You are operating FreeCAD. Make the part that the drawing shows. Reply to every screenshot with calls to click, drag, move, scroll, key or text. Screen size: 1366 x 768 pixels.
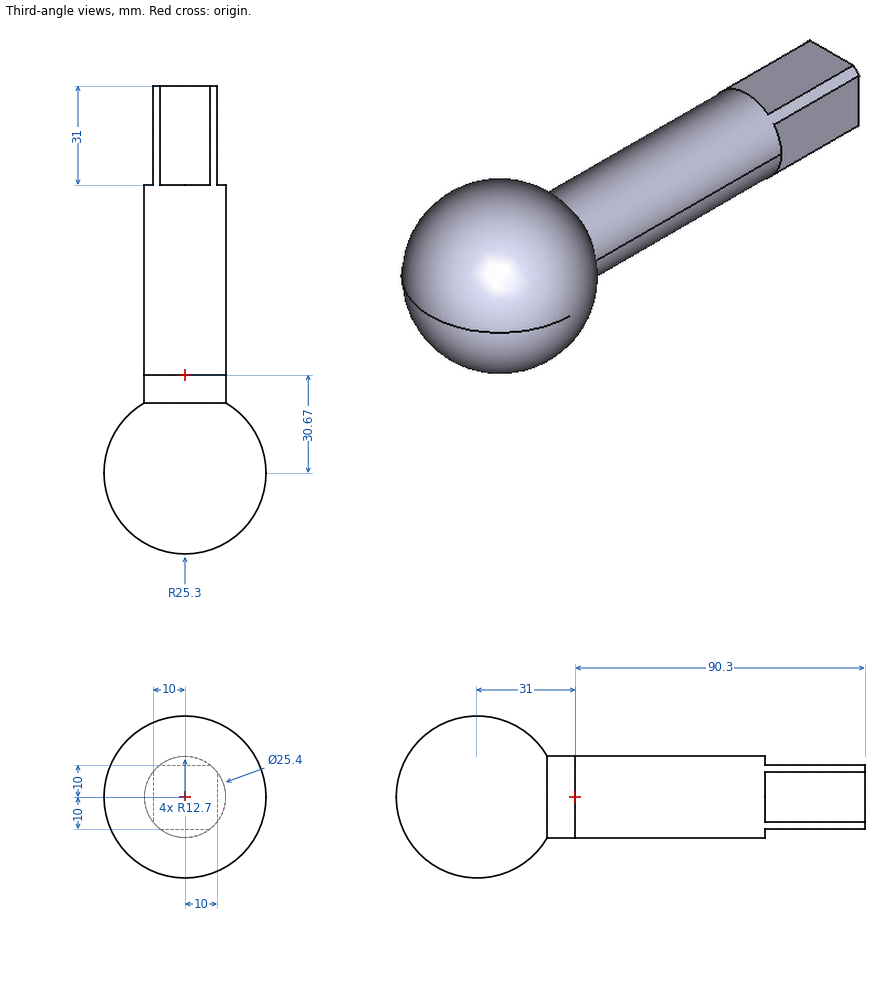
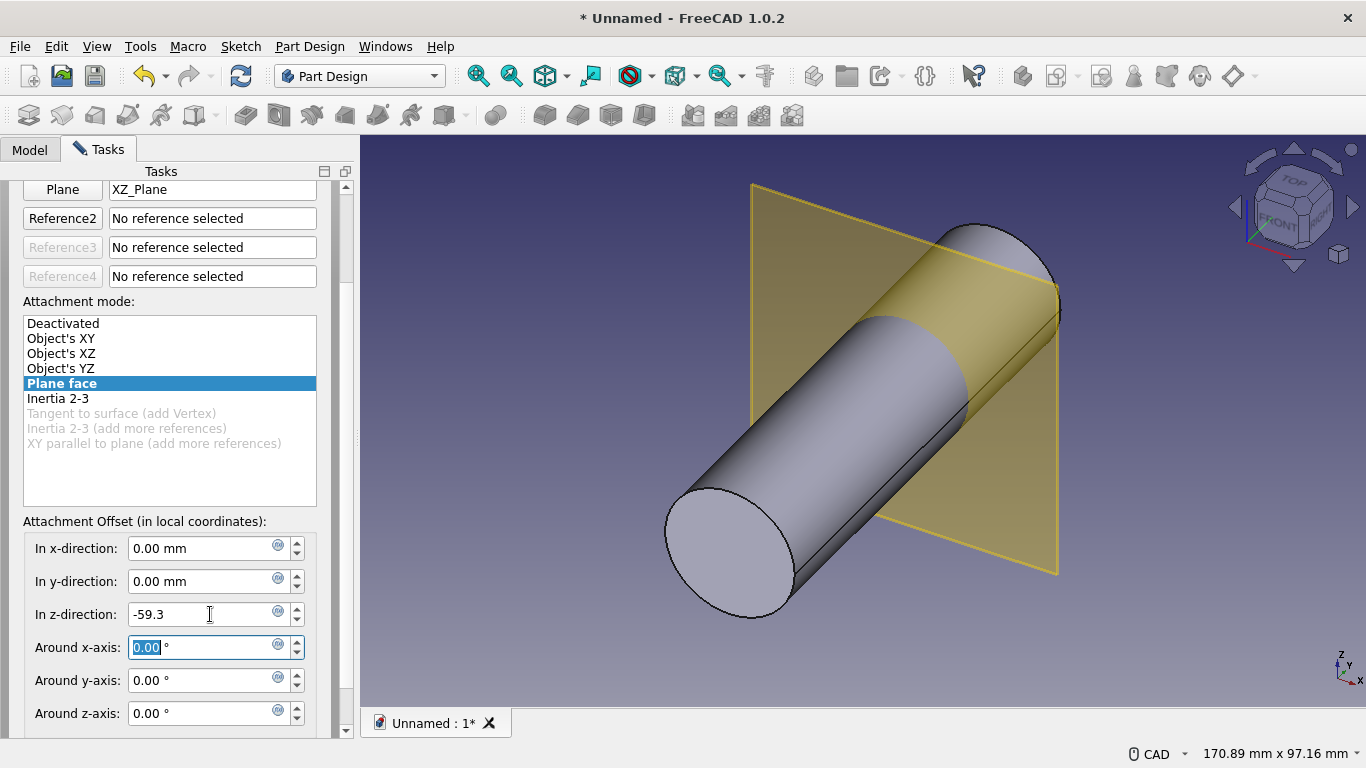
scroll(346, 460, up, 3)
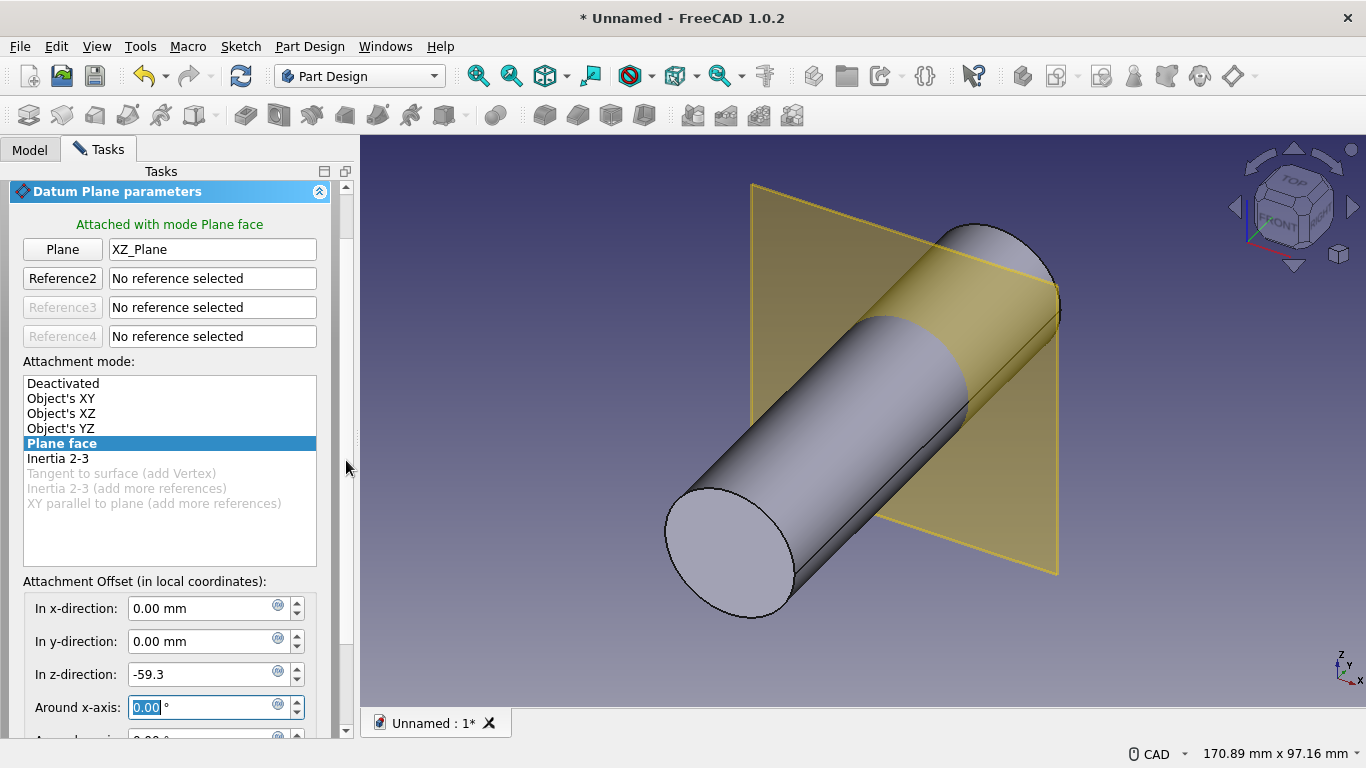
click(127, 210)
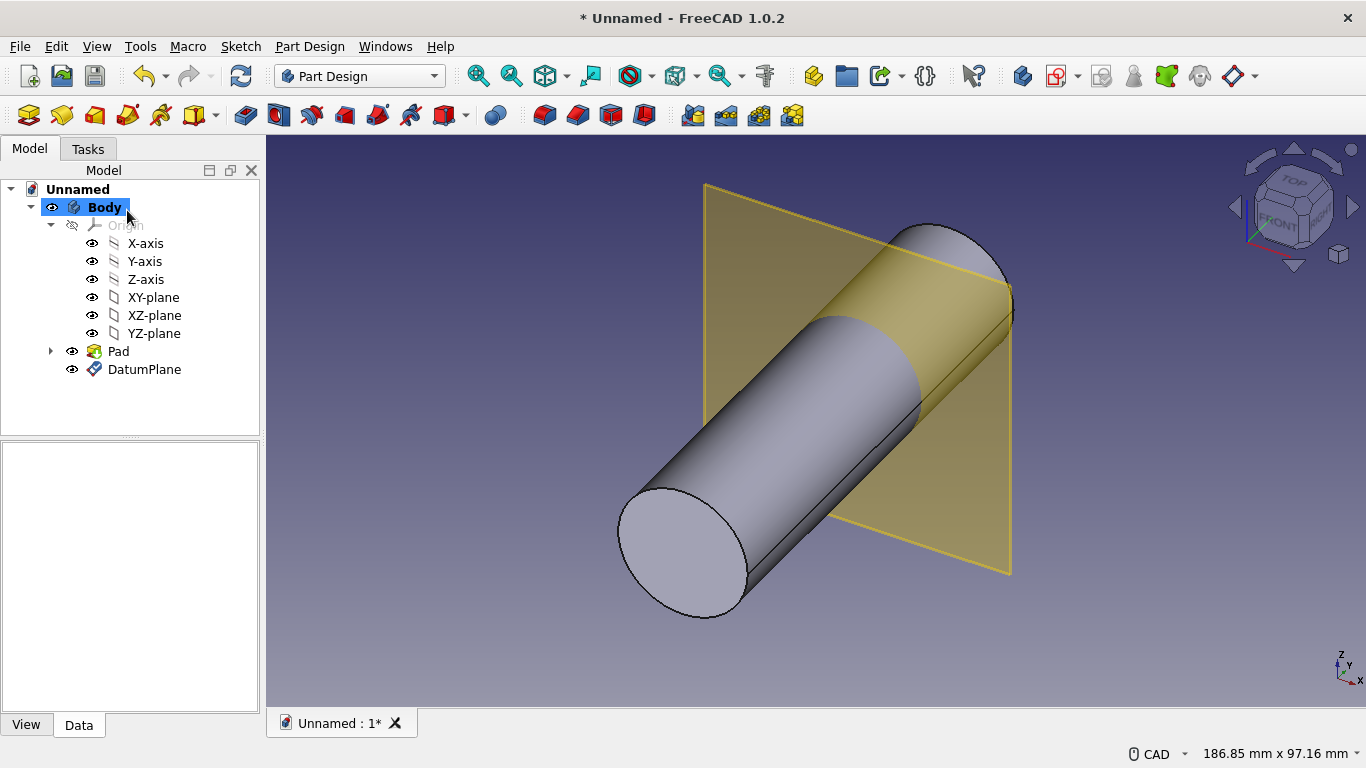
click(117, 369)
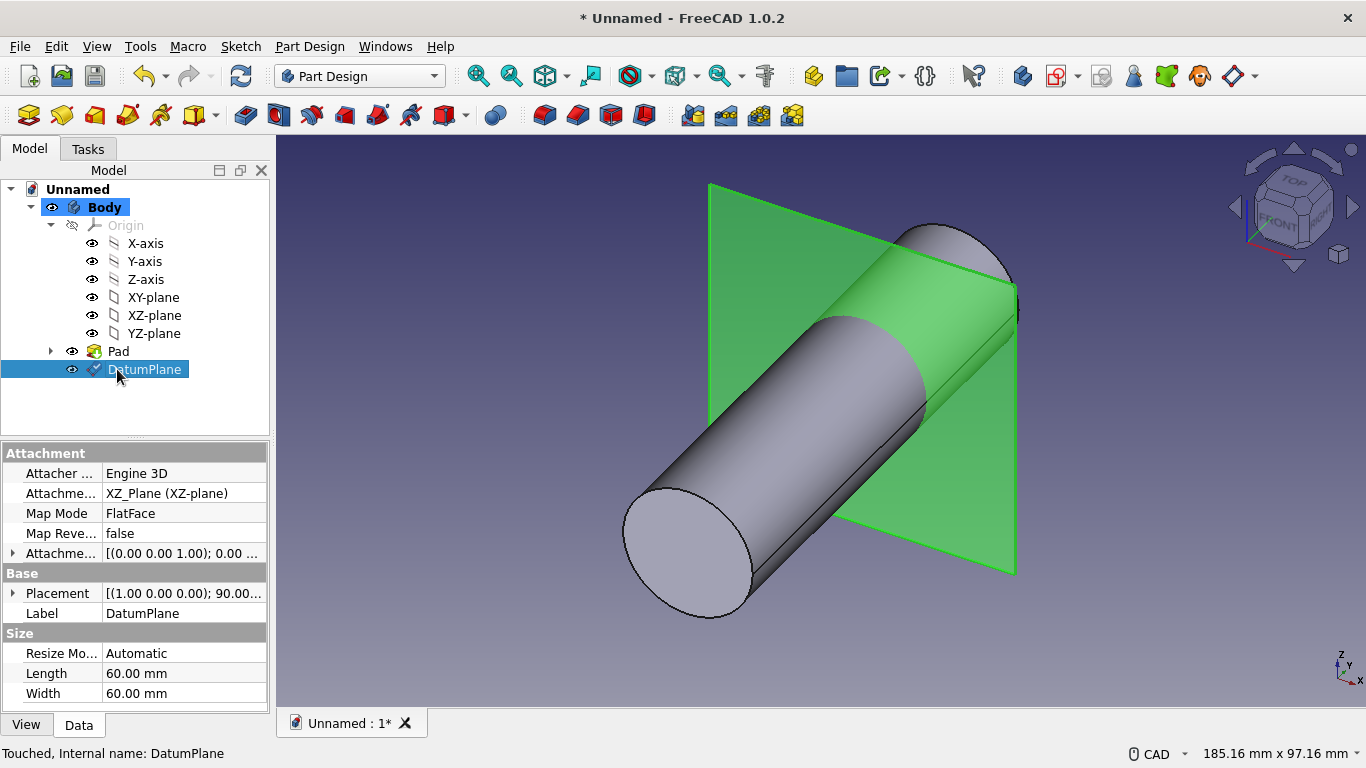
click(1056, 76)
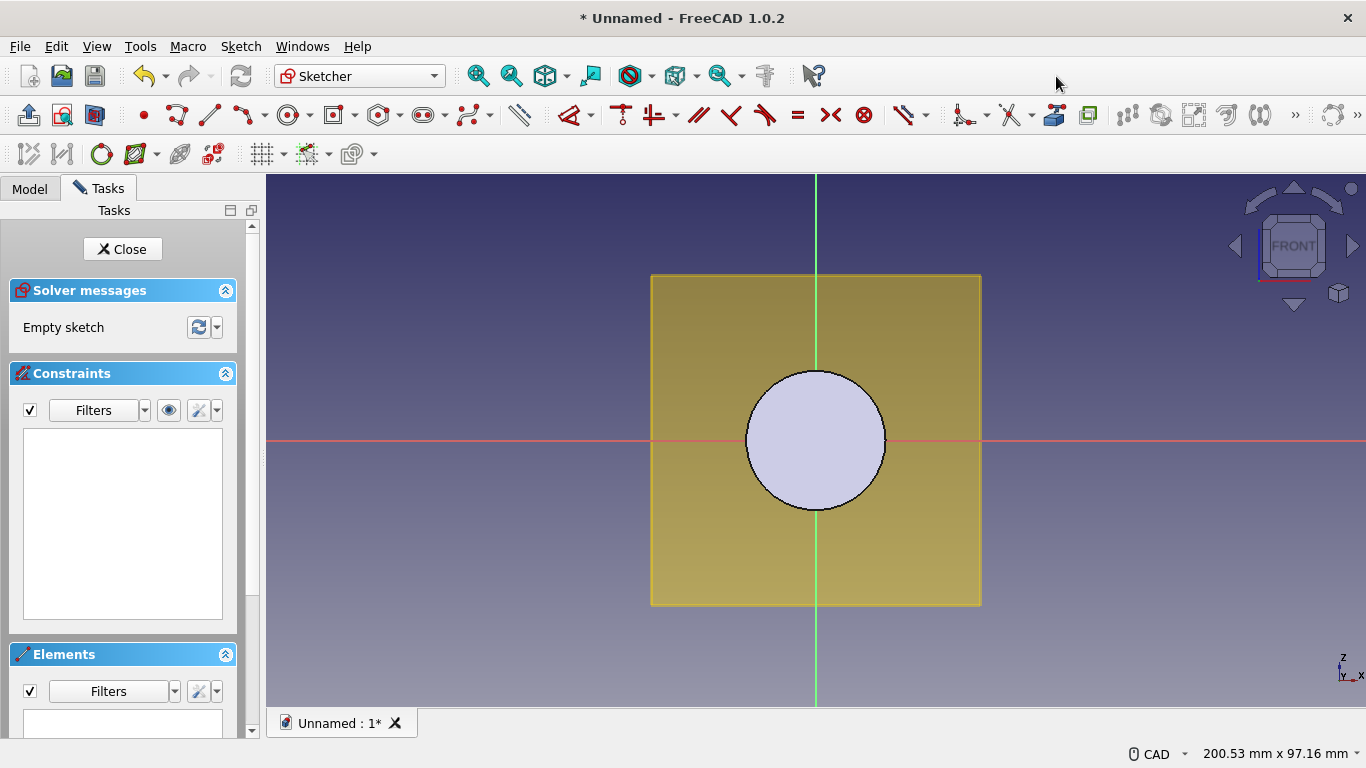
key(q)
key(s)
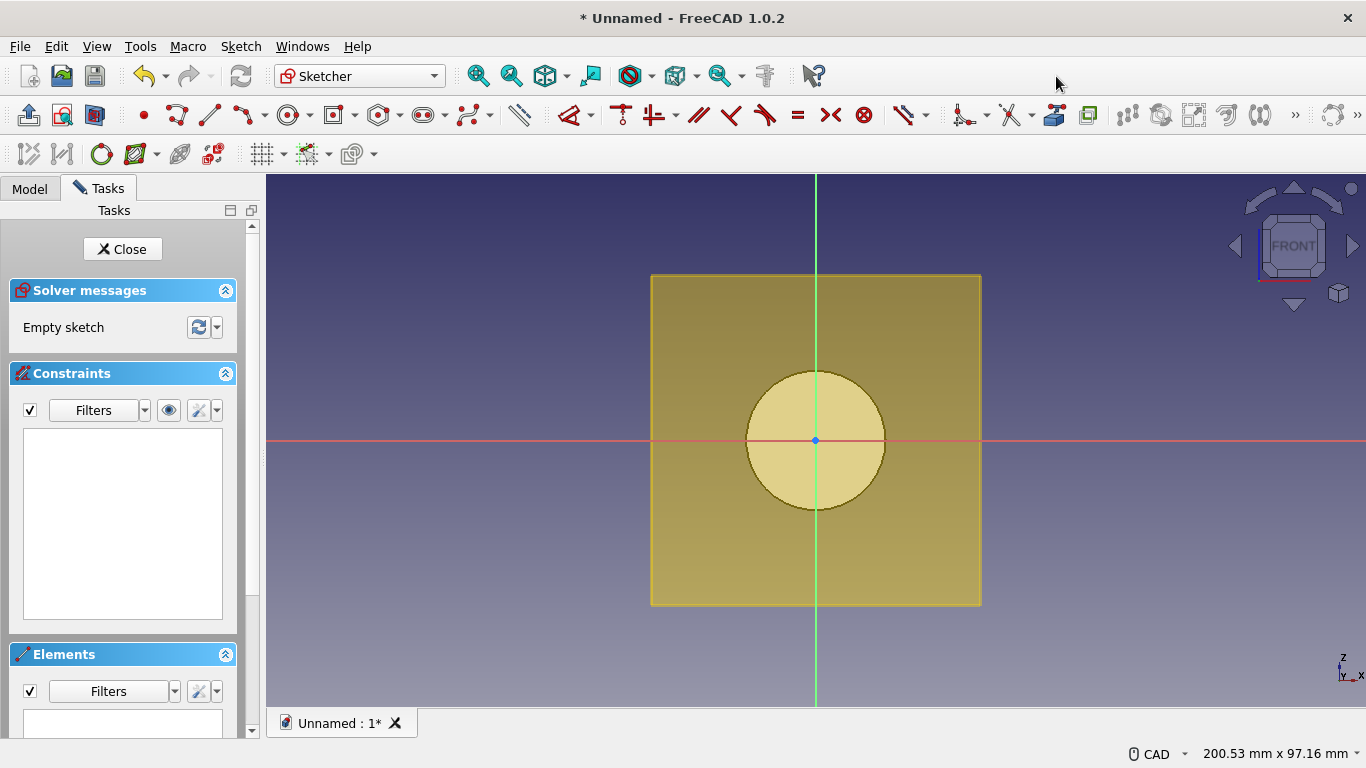
scroll(872, 441, up, 4)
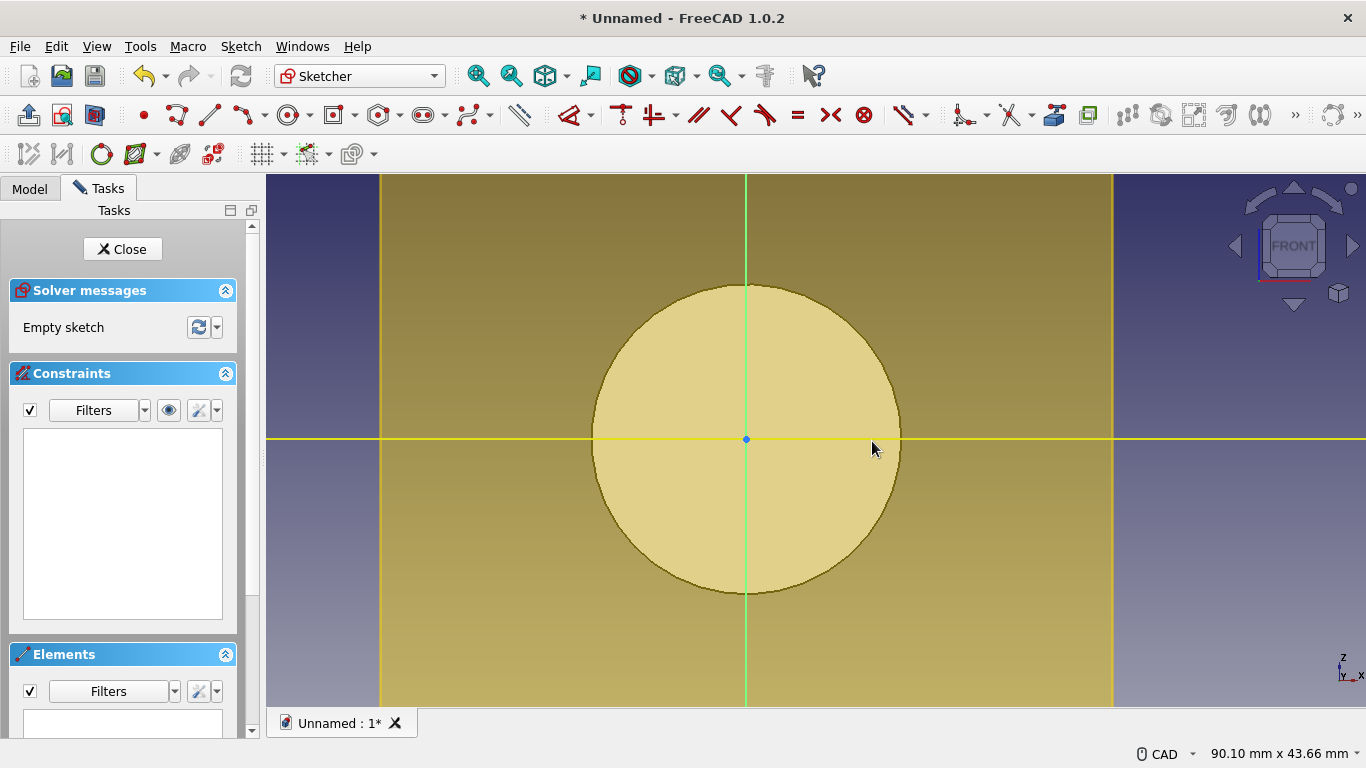
click(210, 116)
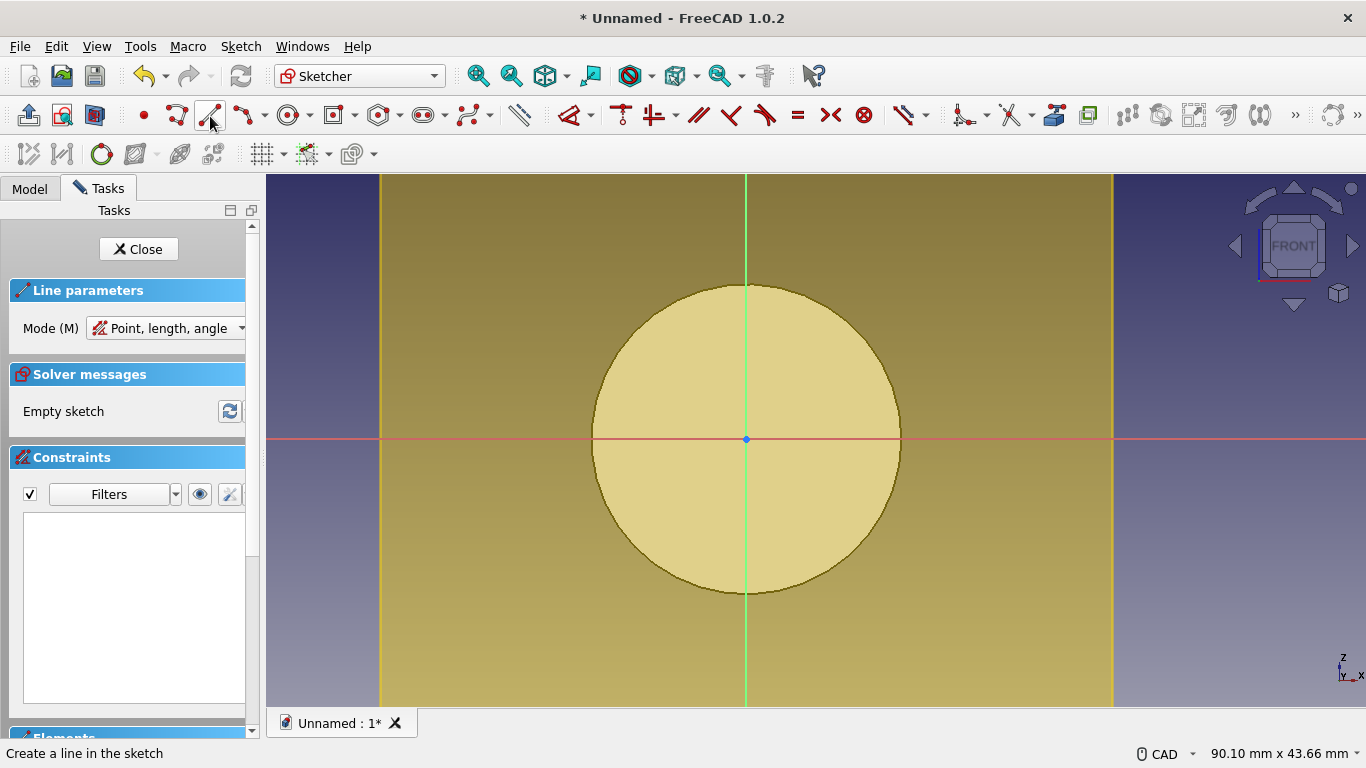
click(651, 317)
click(842, 317)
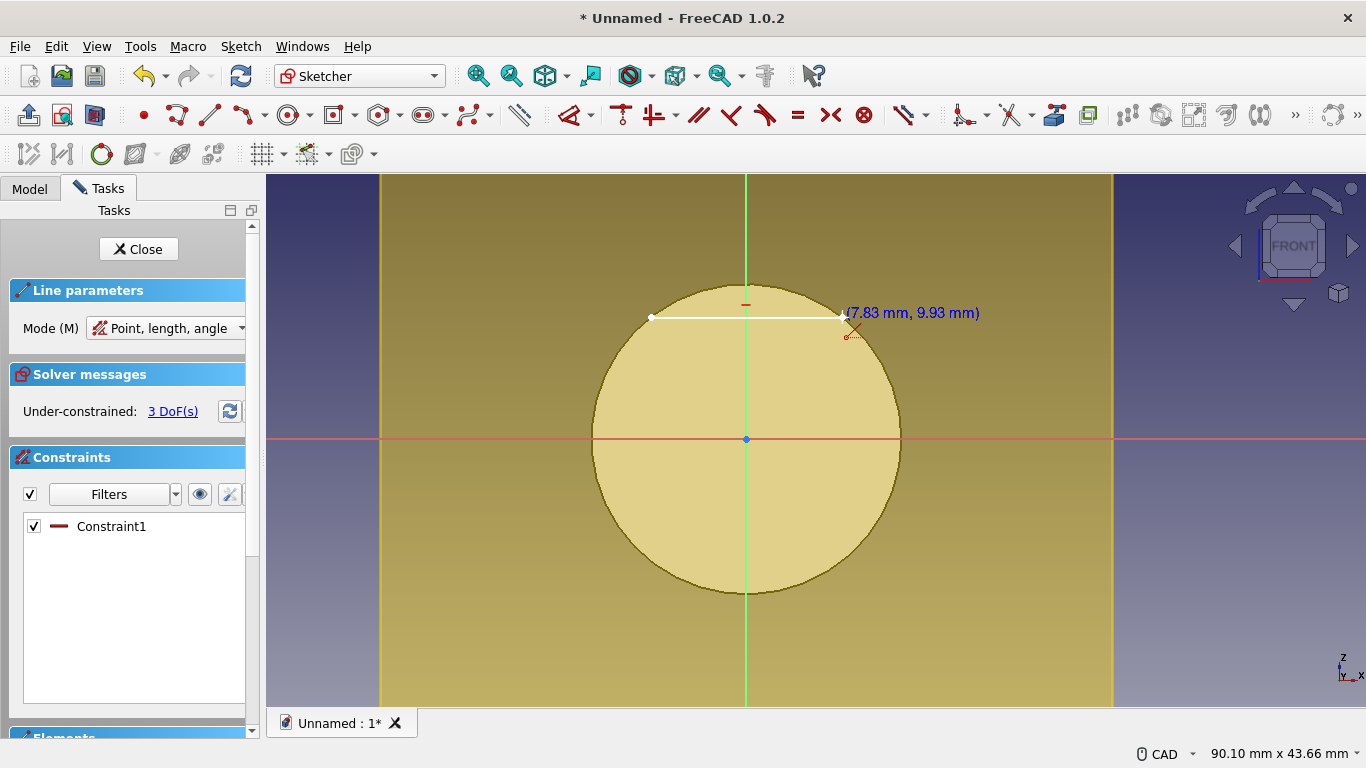
click(242, 116)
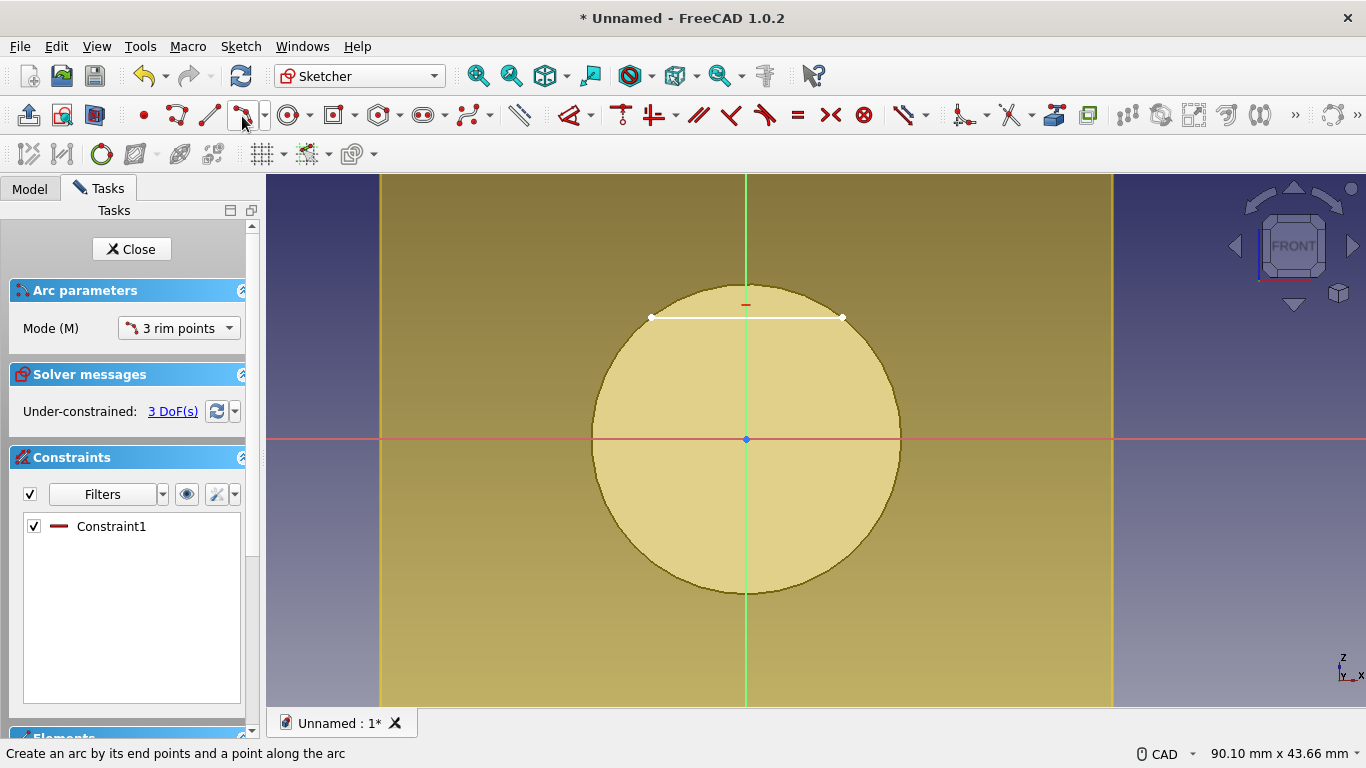
click(842, 318)
click(651, 318)
click(767, 286)